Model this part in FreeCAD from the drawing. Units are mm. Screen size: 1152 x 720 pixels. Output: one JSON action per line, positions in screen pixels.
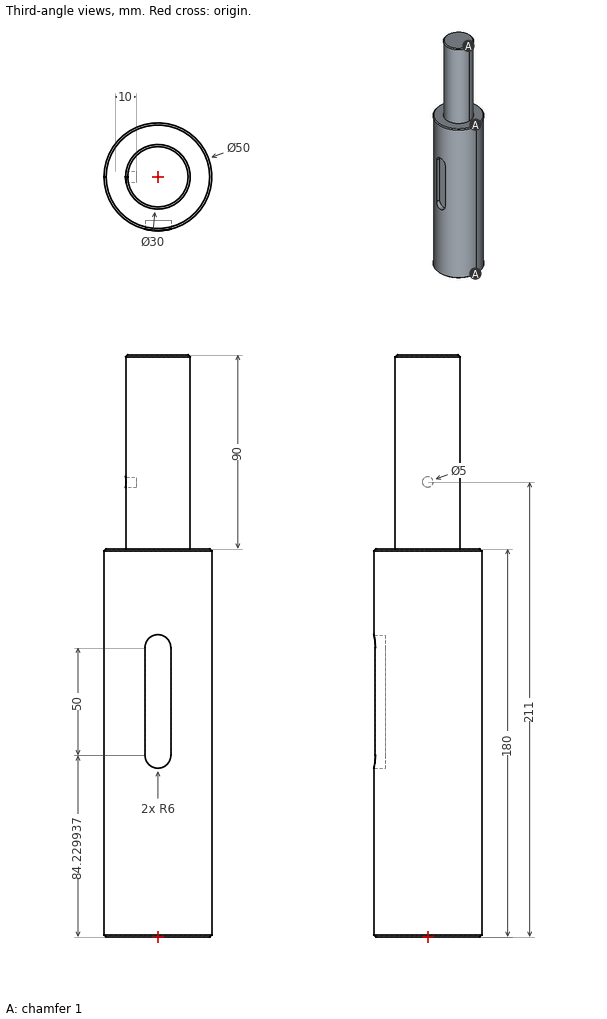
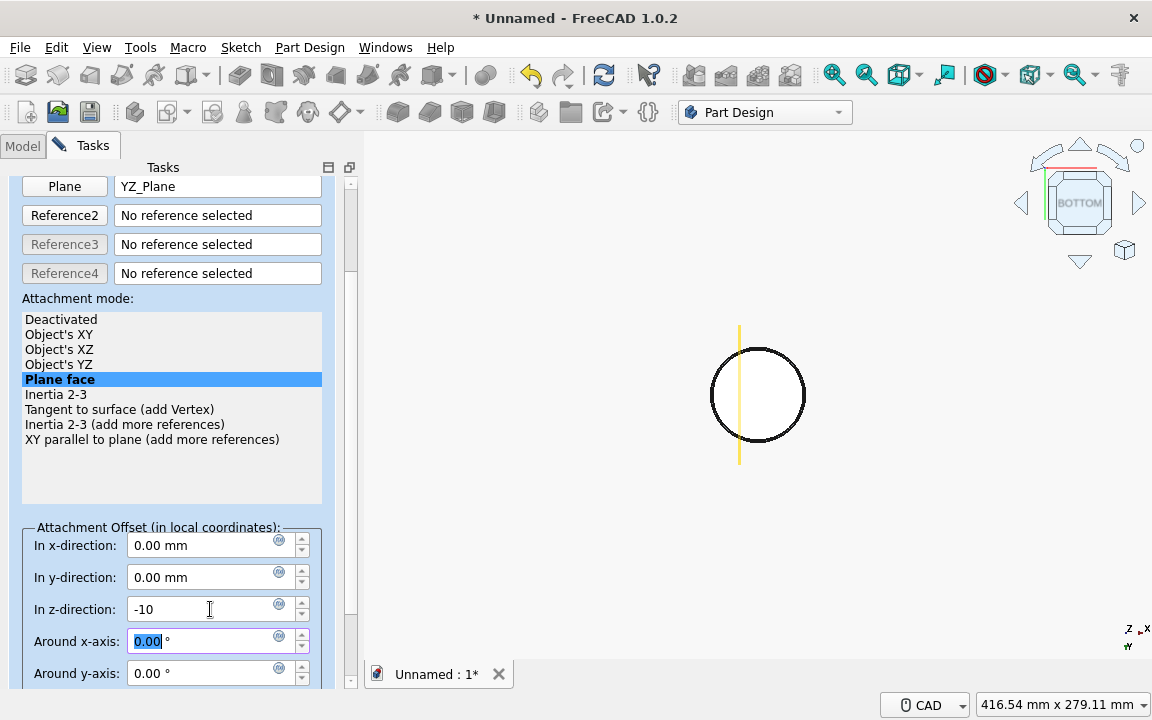
{"action": "scroll", "coordinate": [351, 432], "scroll_direction": "up", "scroll_amount": 3}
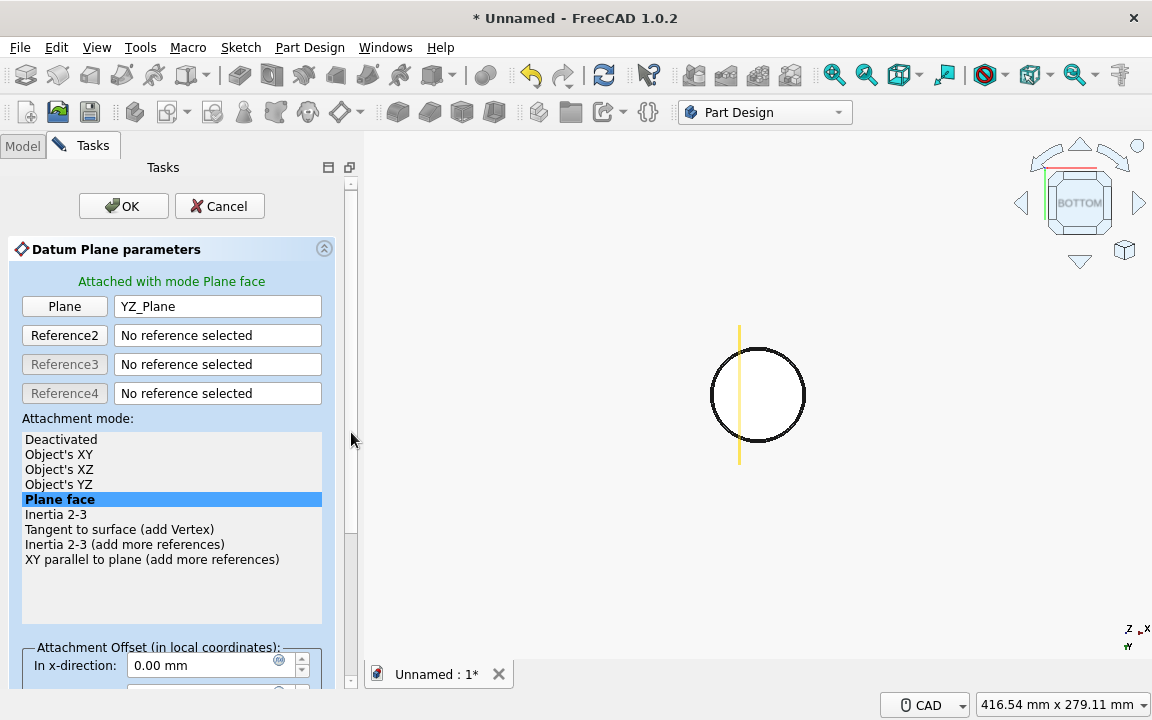
{"action": "left_click", "coordinate": [124, 206]}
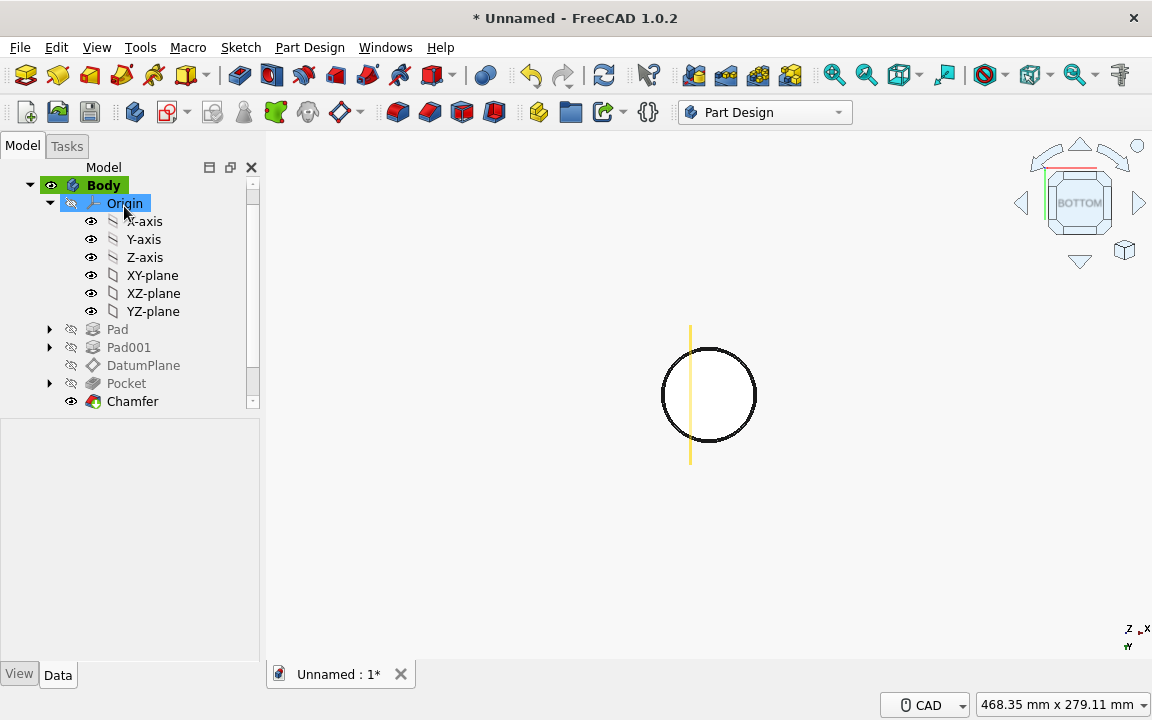
{"action": "scroll", "coordinate": [120, 289], "scroll_direction": "down", "scroll_amount": 3}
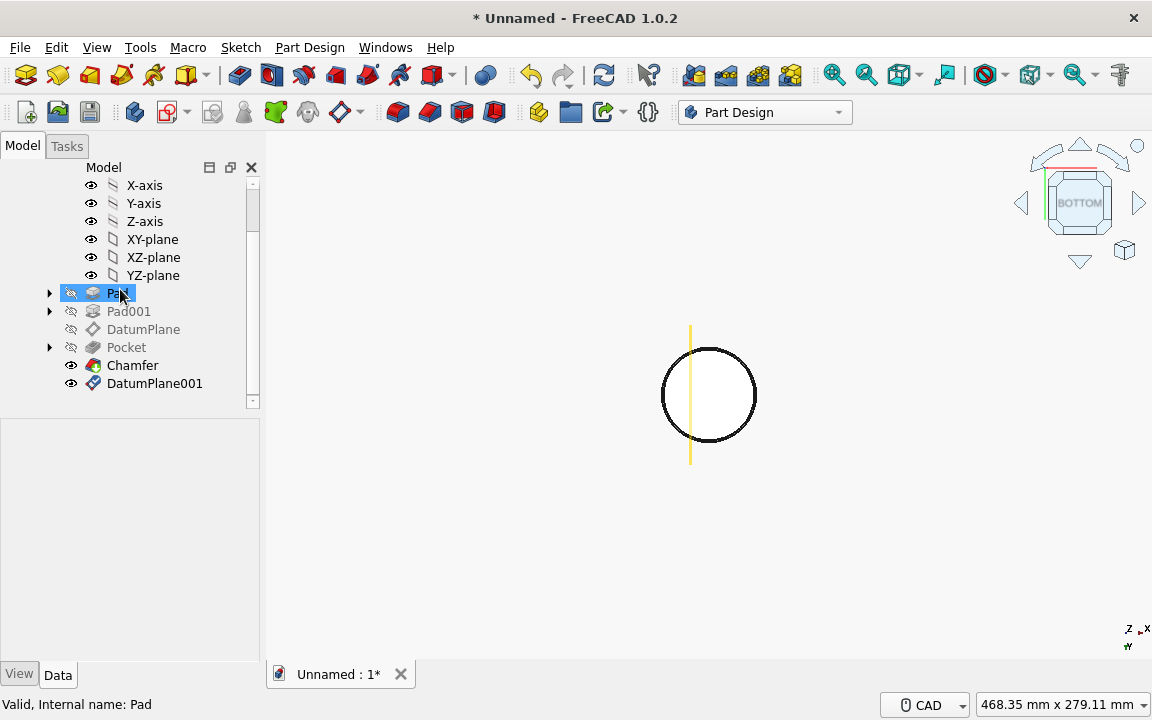
{"action": "left_click", "coordinate": [116, 383]}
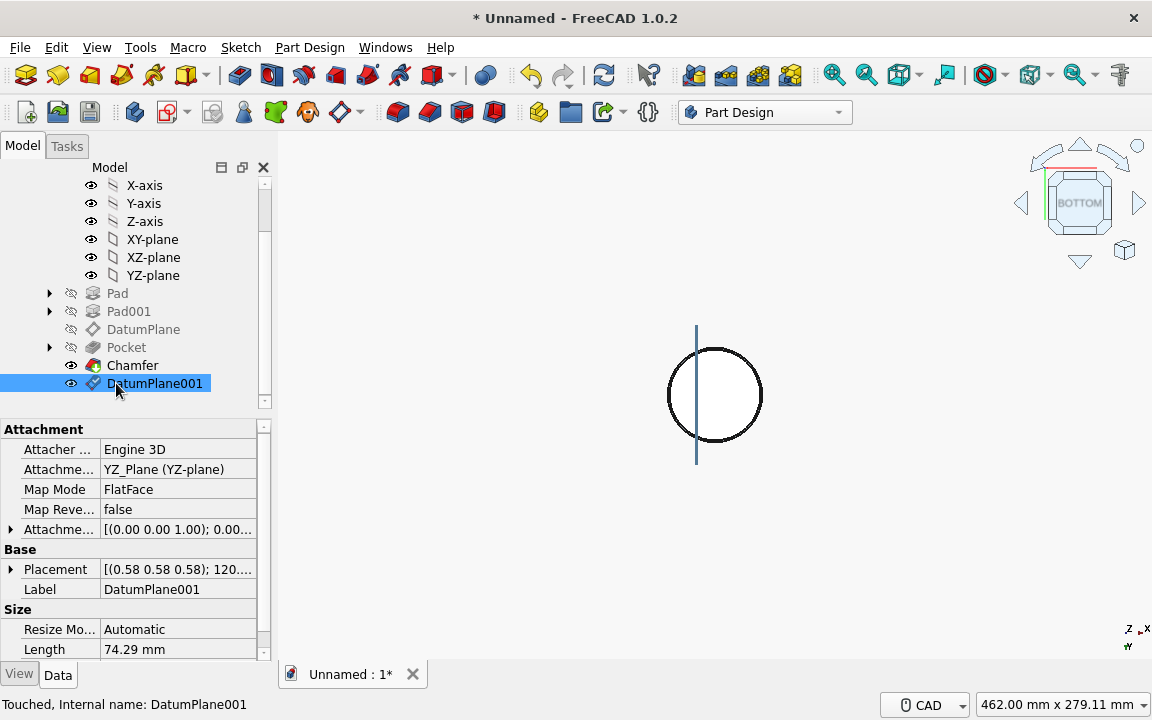
{"action": "left_click", "coordinate": [168, 112]}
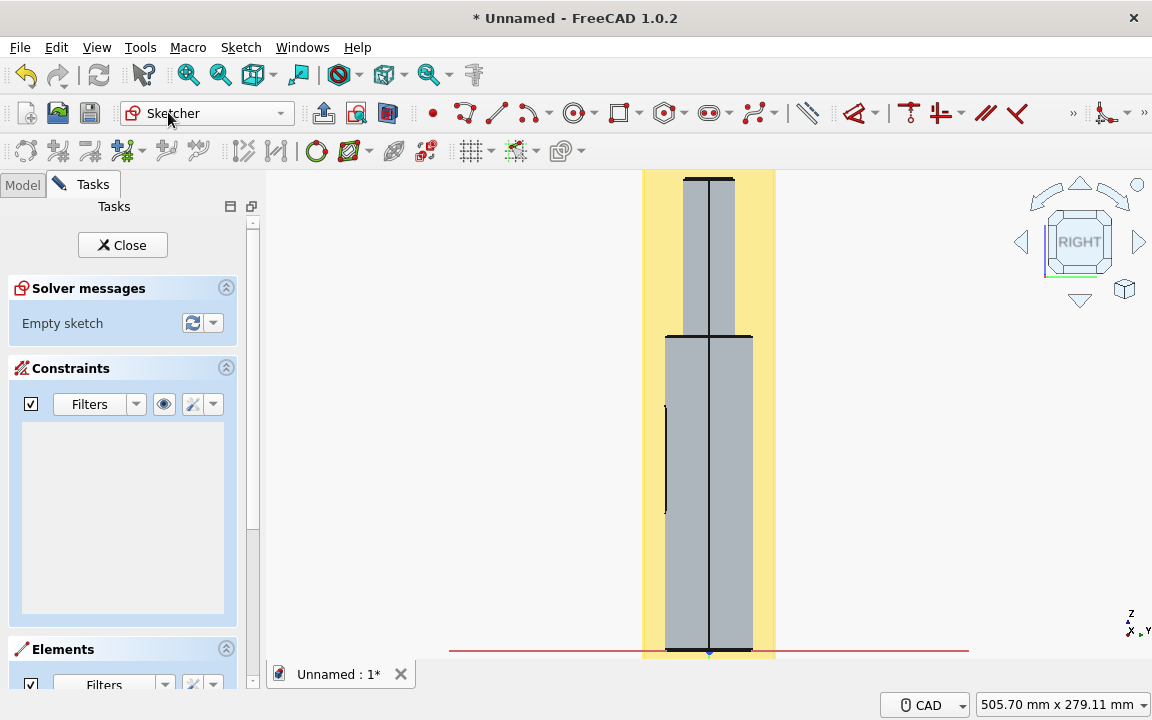
{"action": "key", "text": "q s"}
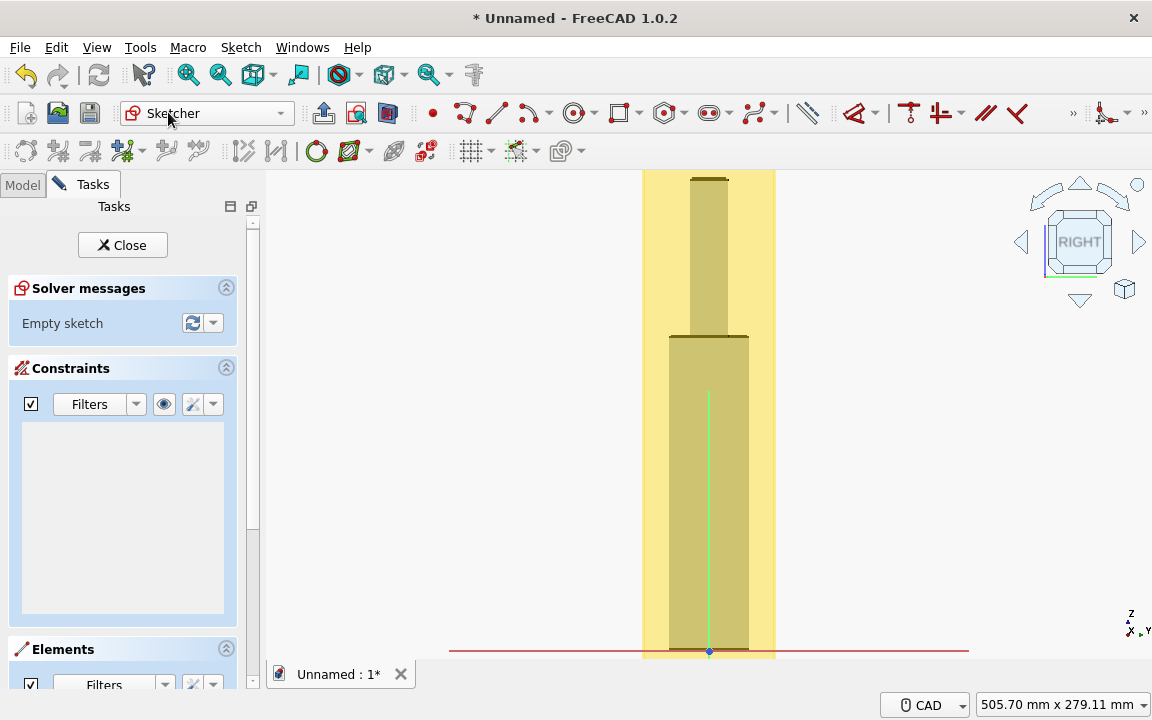
{"action": "scroll", "coordinate": [713, 274], "scroll_direction": "up", "scroll_amount": 15}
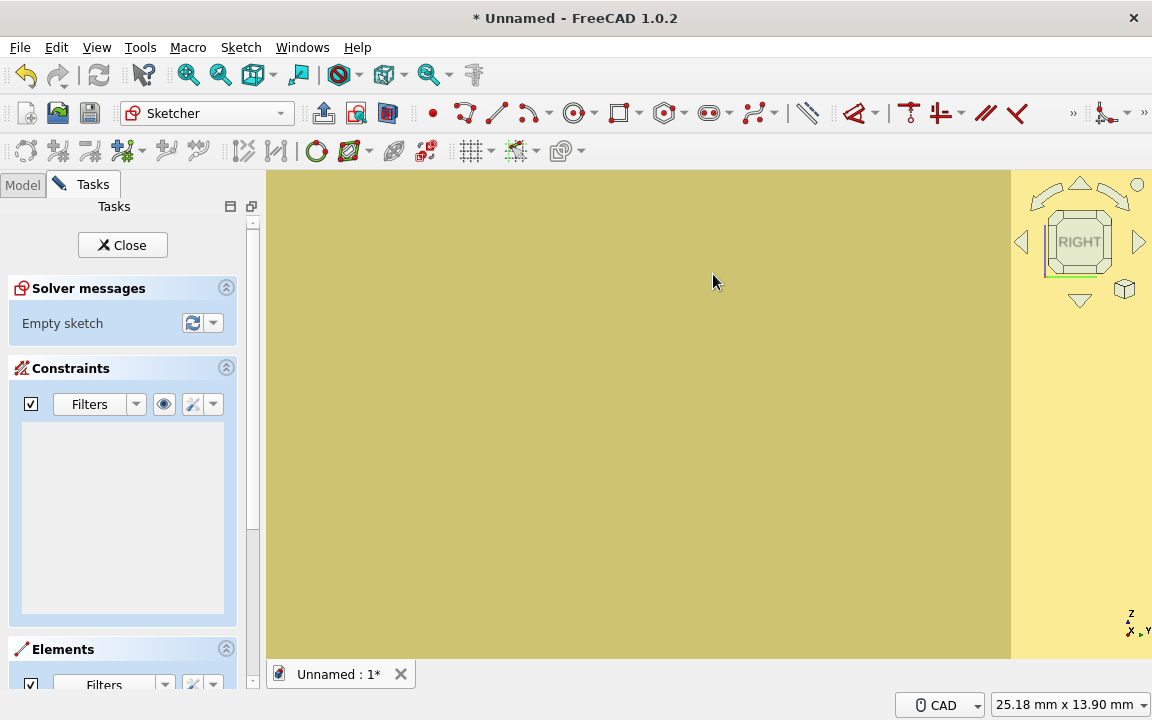
{"action": "scroll", "coordinate": [602, 421], "scroll_direction": "up", "scroll_amount": 3}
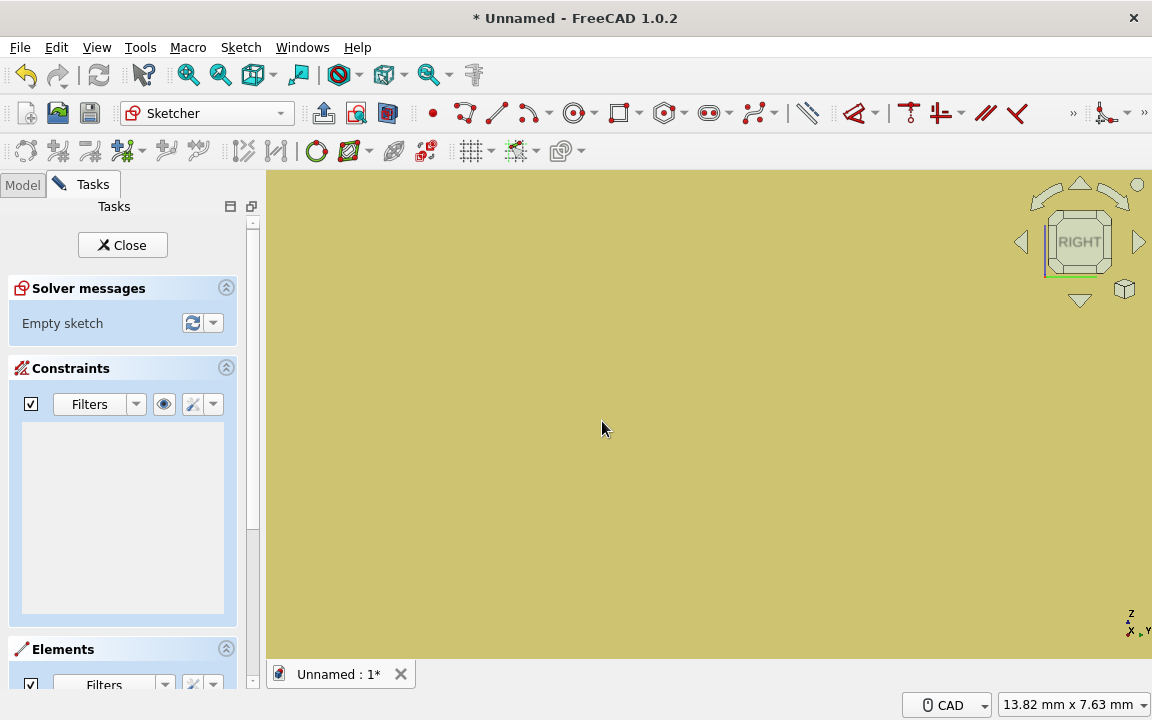
{"action": "key", "text": "g c"}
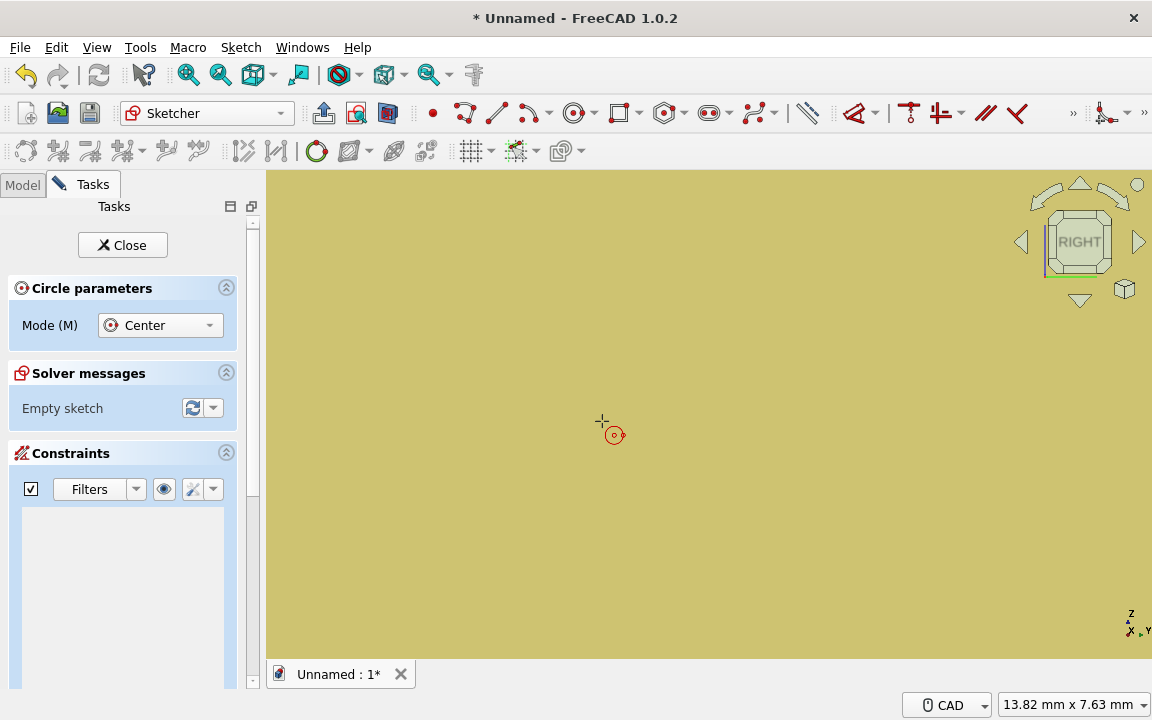
{"action": "left_click", "coordinate": [640, 414]}
{"action": "left_click", "coordinate": [753, 301]}
{"action": "key", "text": "Escape"}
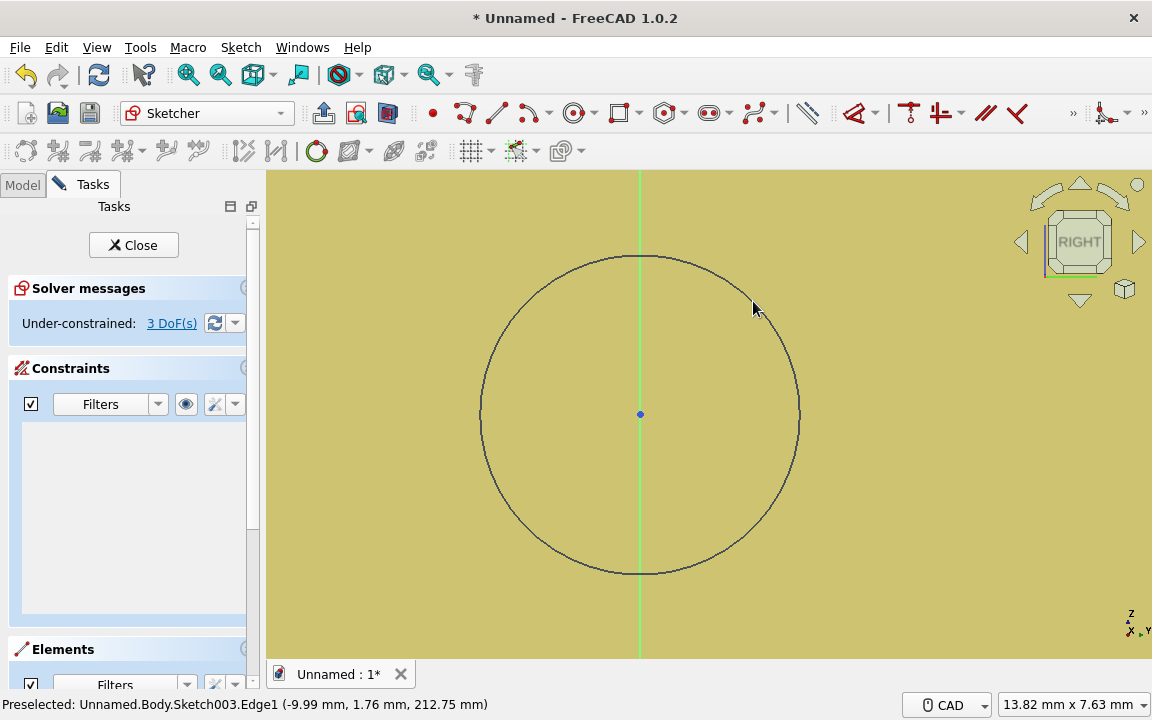
{"action": "left_click", "coordinate": [640, 415]}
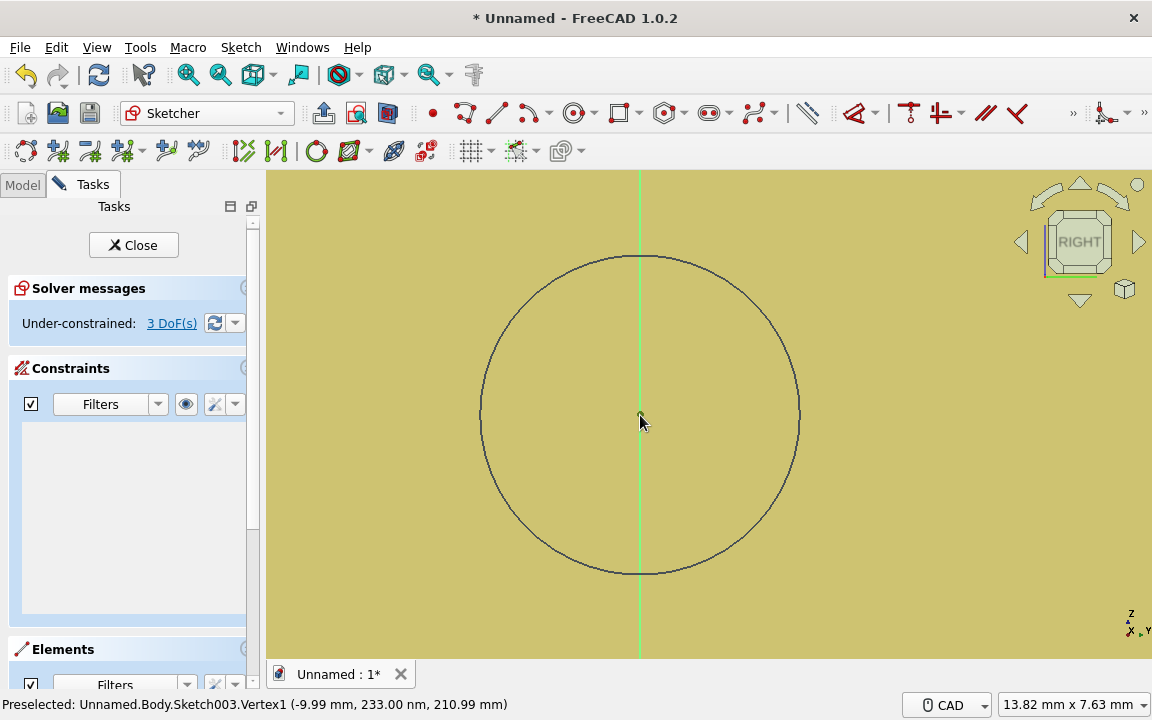
{"action": "left_click", "coordinate": [640, 538]}